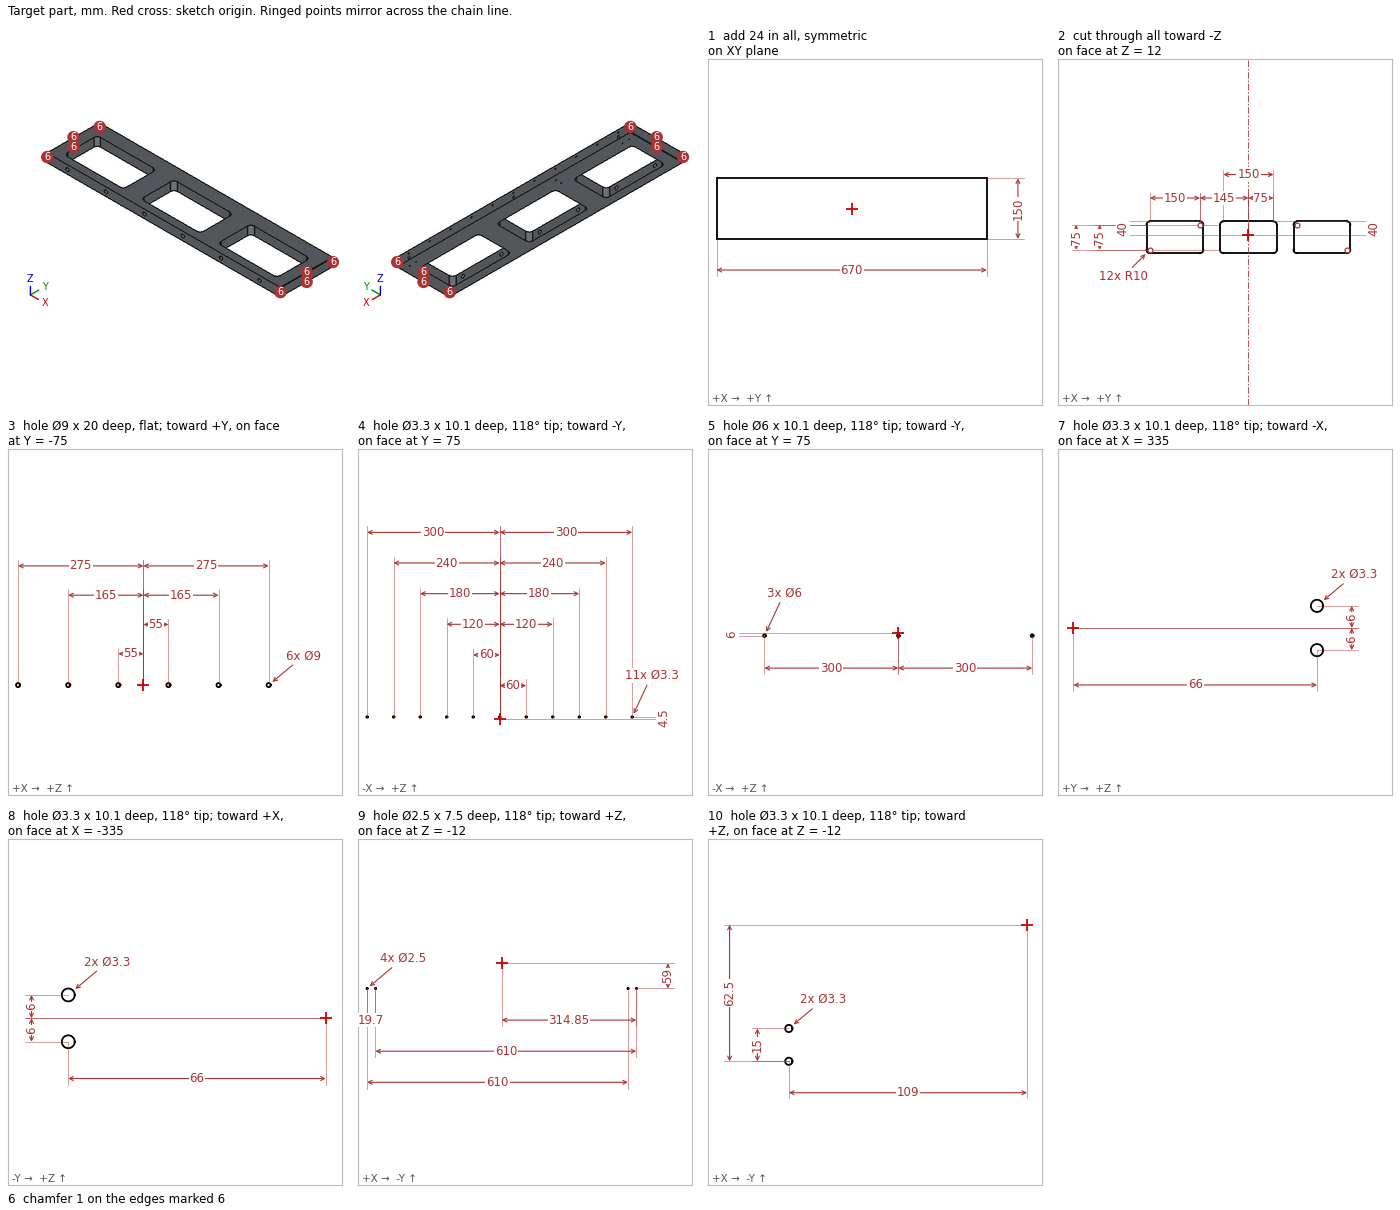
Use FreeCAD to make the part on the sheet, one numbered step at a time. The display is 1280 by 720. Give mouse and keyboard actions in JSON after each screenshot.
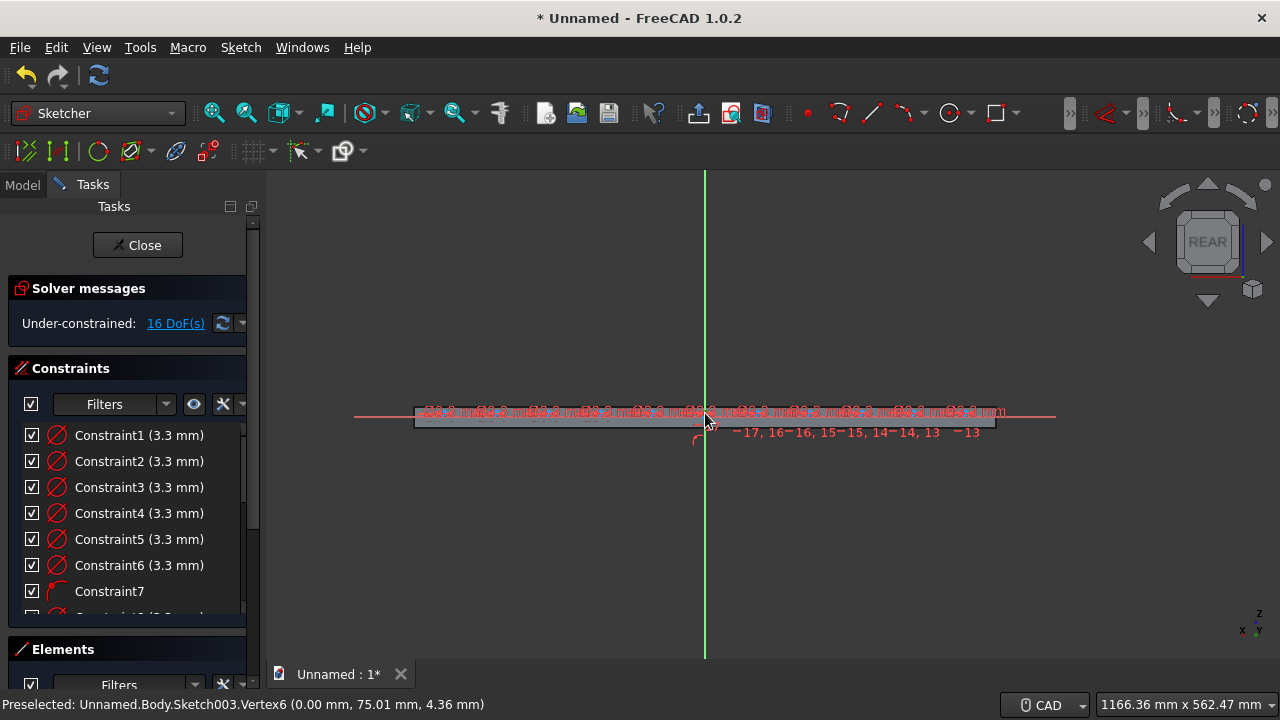
{"action": "left_click", "coordinate": [653, 413]}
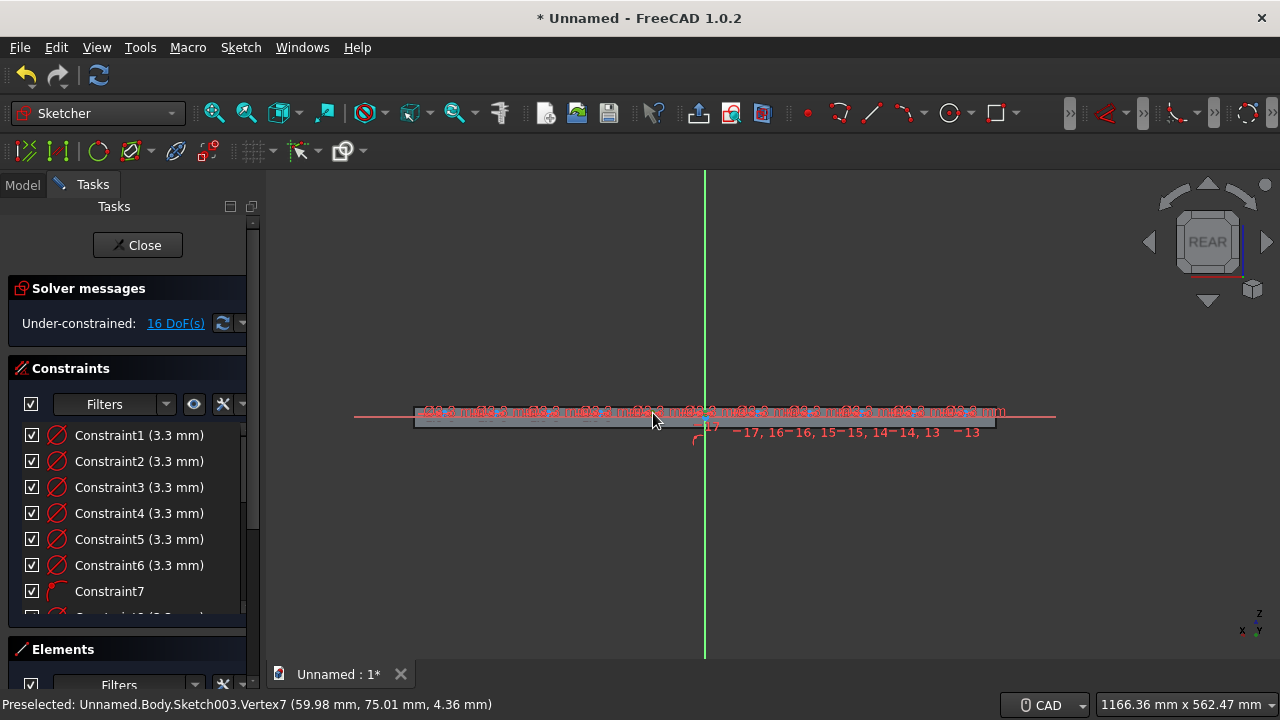
{"action": "key", "text": "h"}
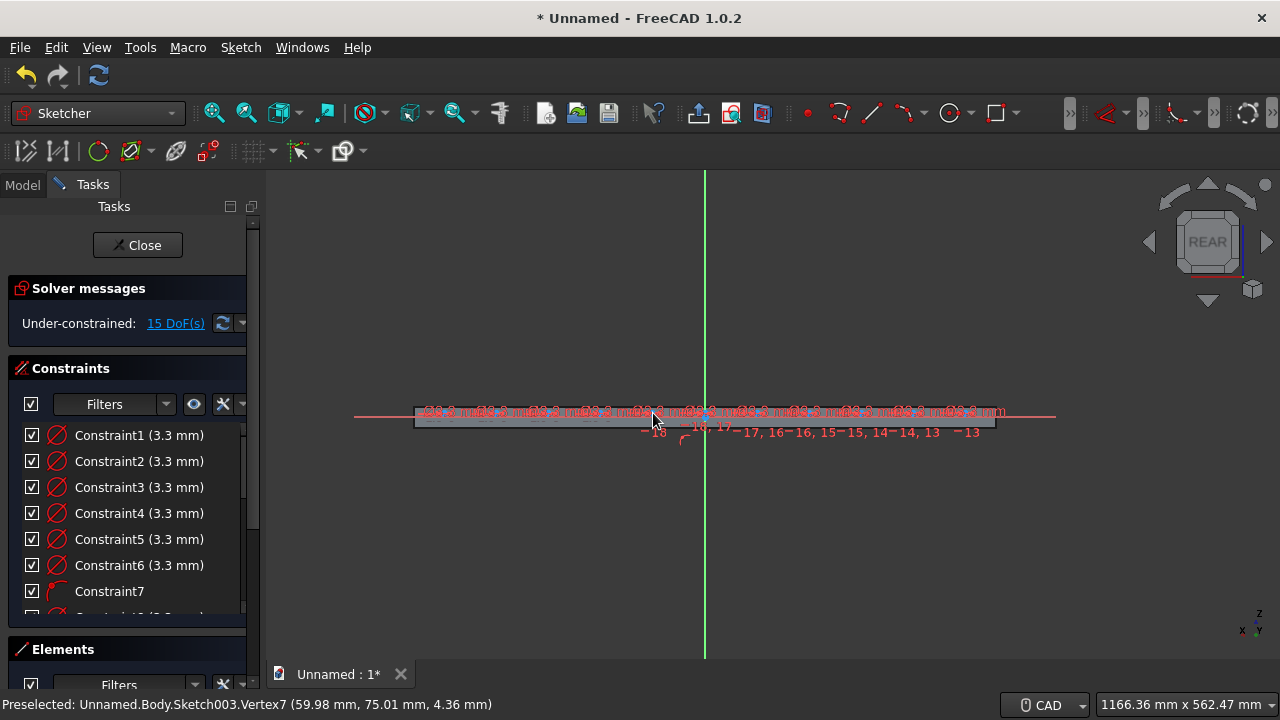
{"action": "left_click", "coordinate": [653, 413]}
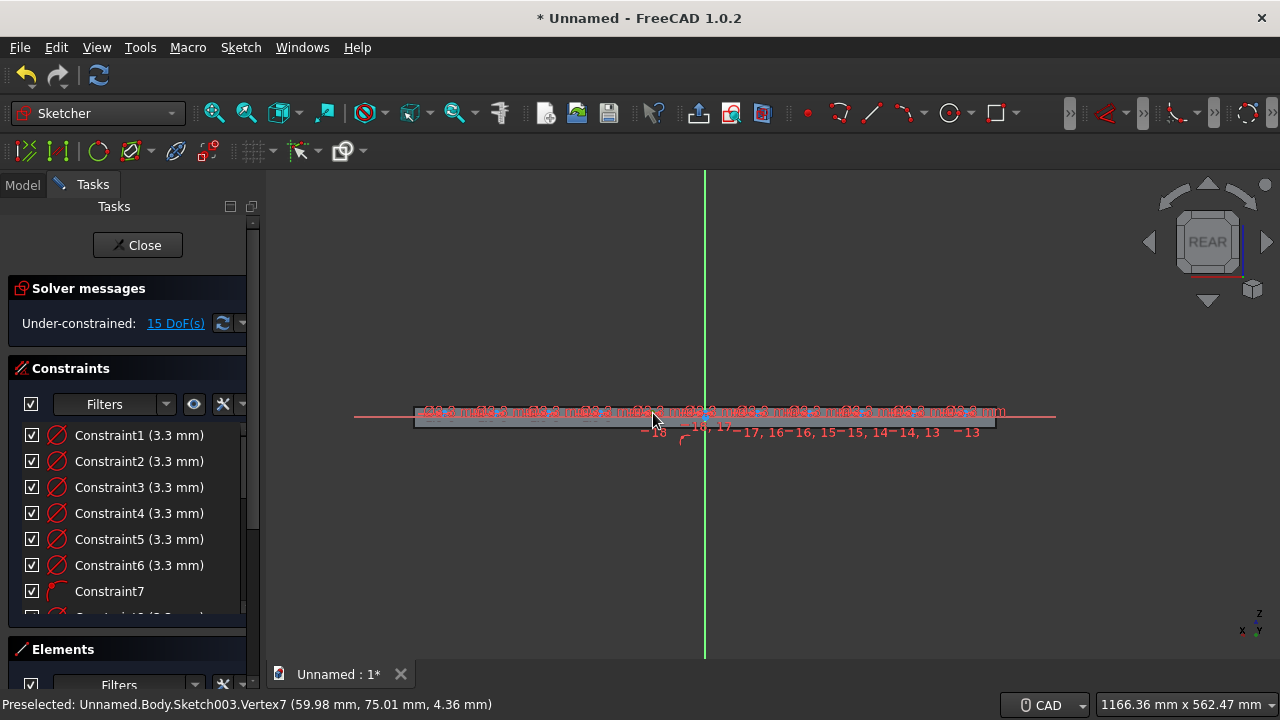
{"action": "left_click", "coordinate": [601, 414]}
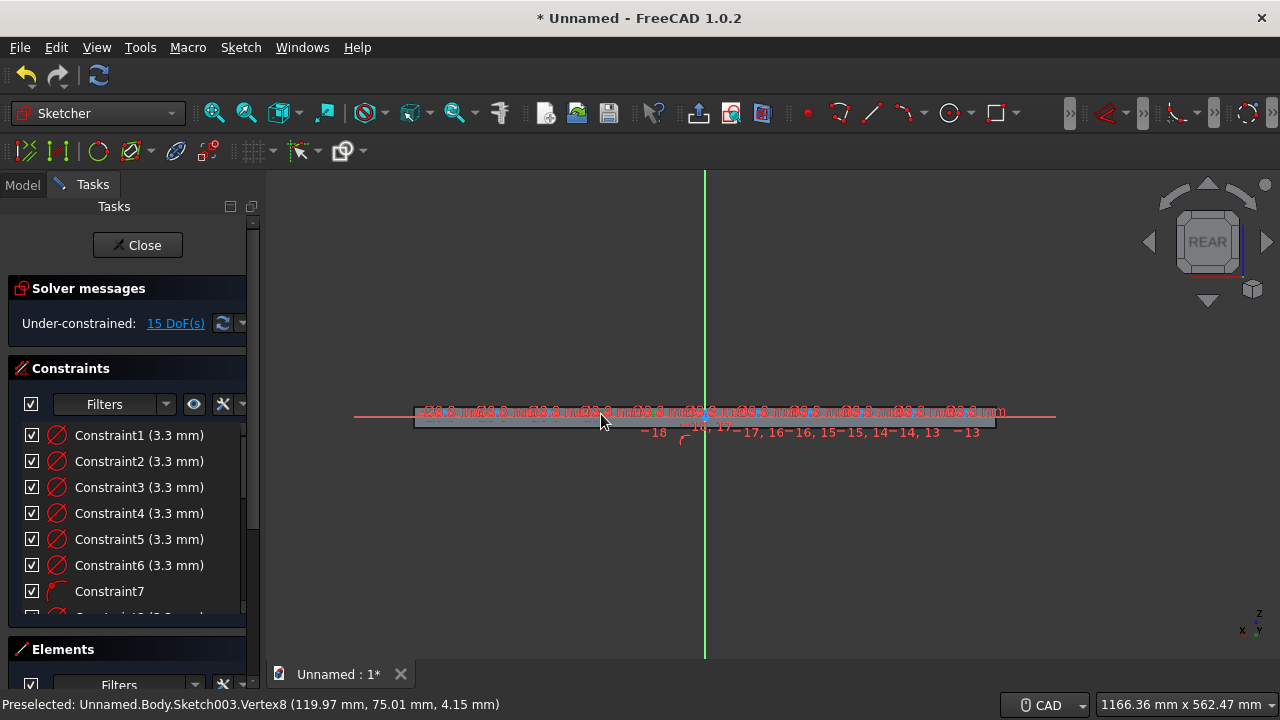
{"action": "key", "text": "h"}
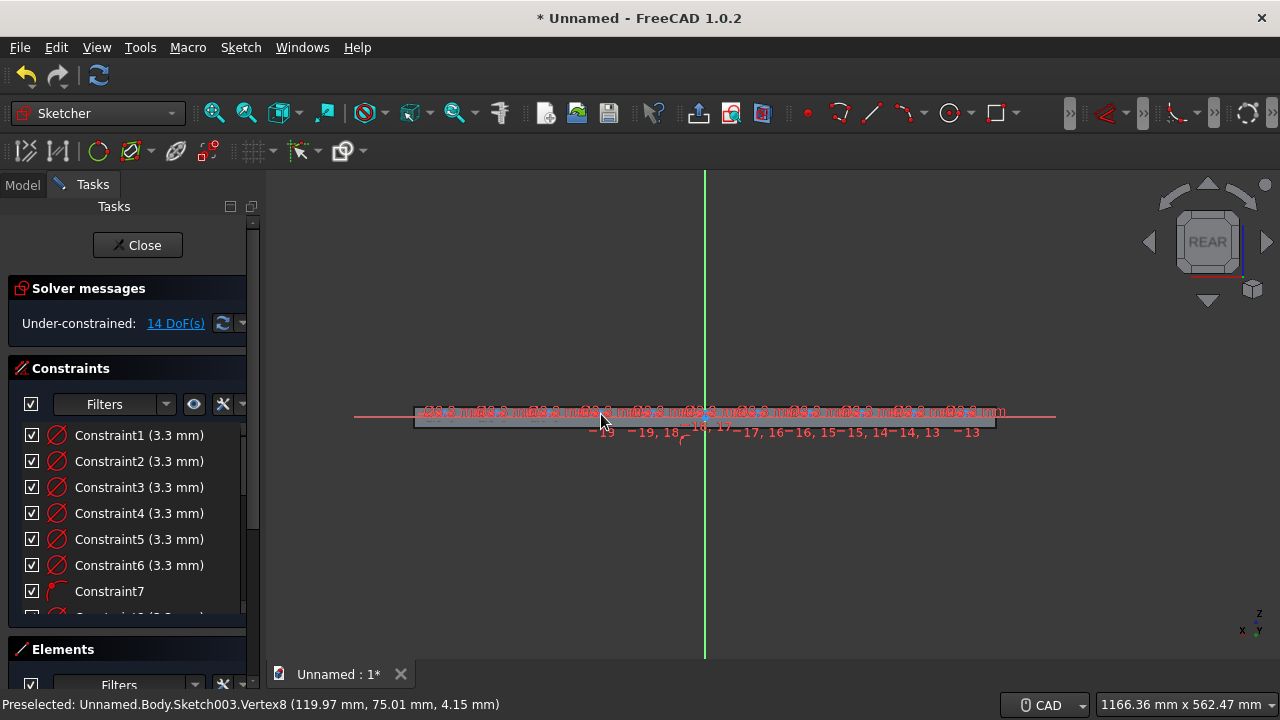
{"action": "left_click", "coordinate": [601, 413]}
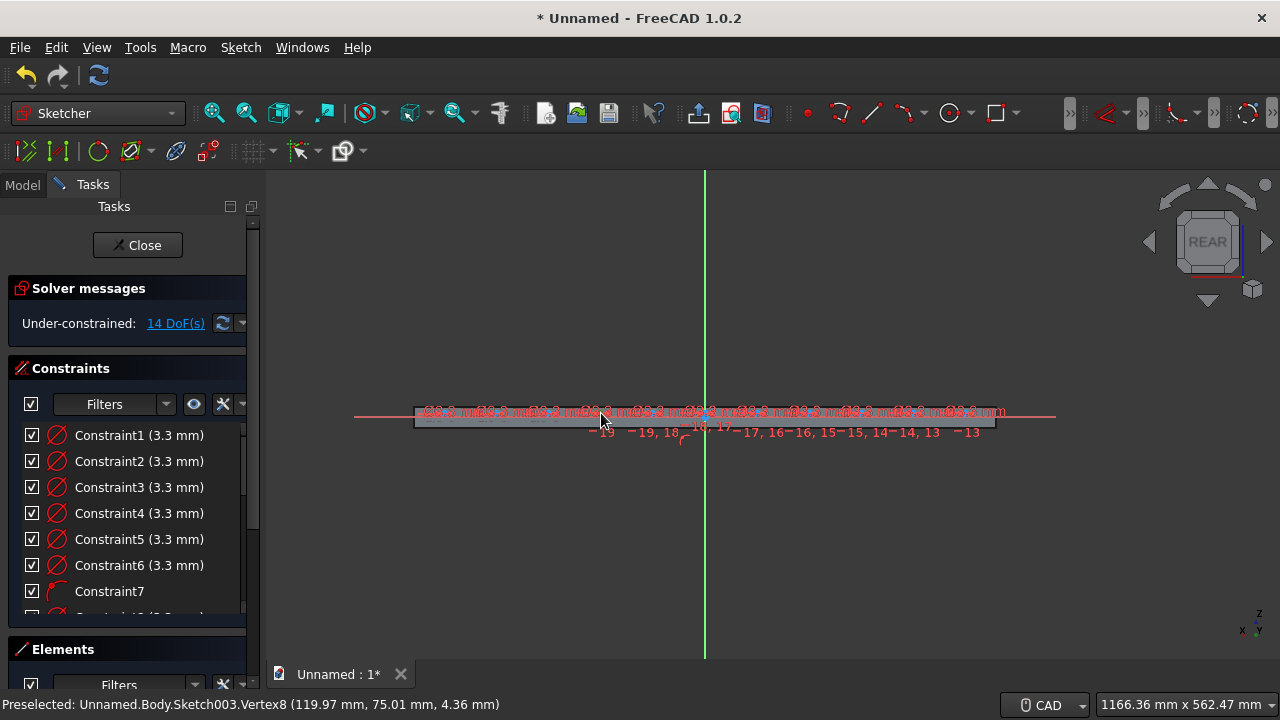
{"action": "left_click", "coordinate": [549, 414]}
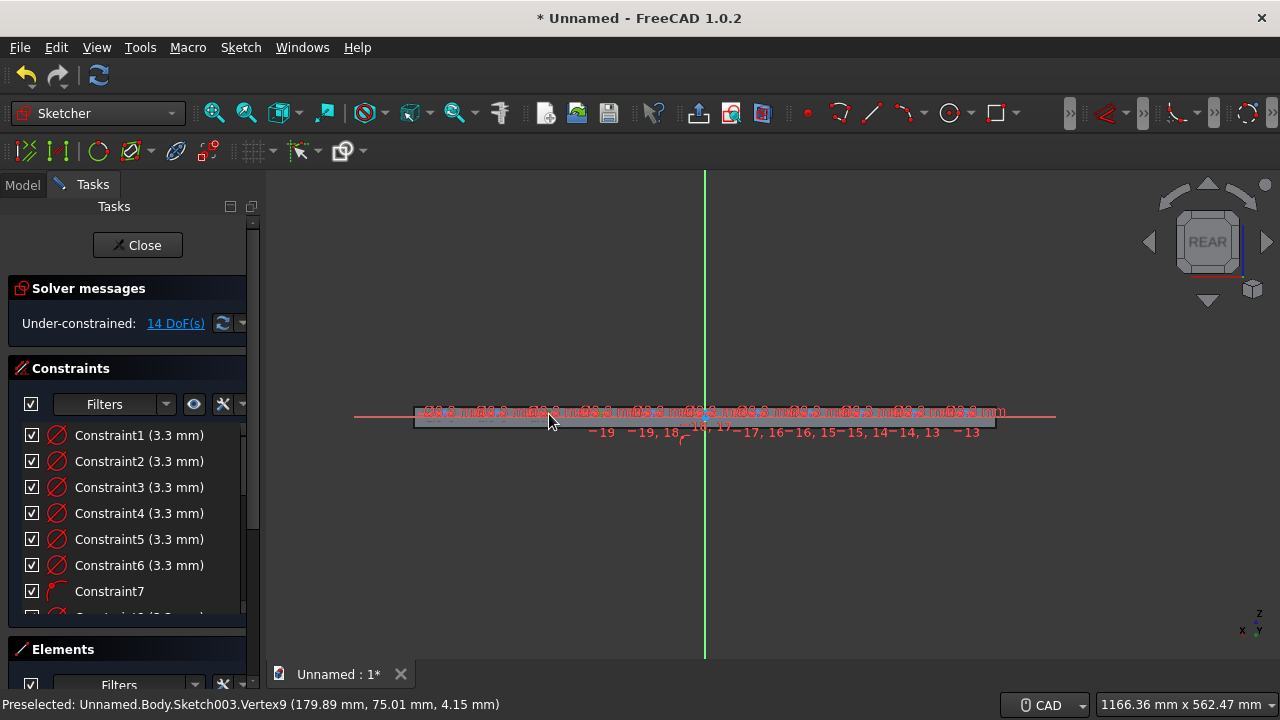
{"action": "key", "text": "h"}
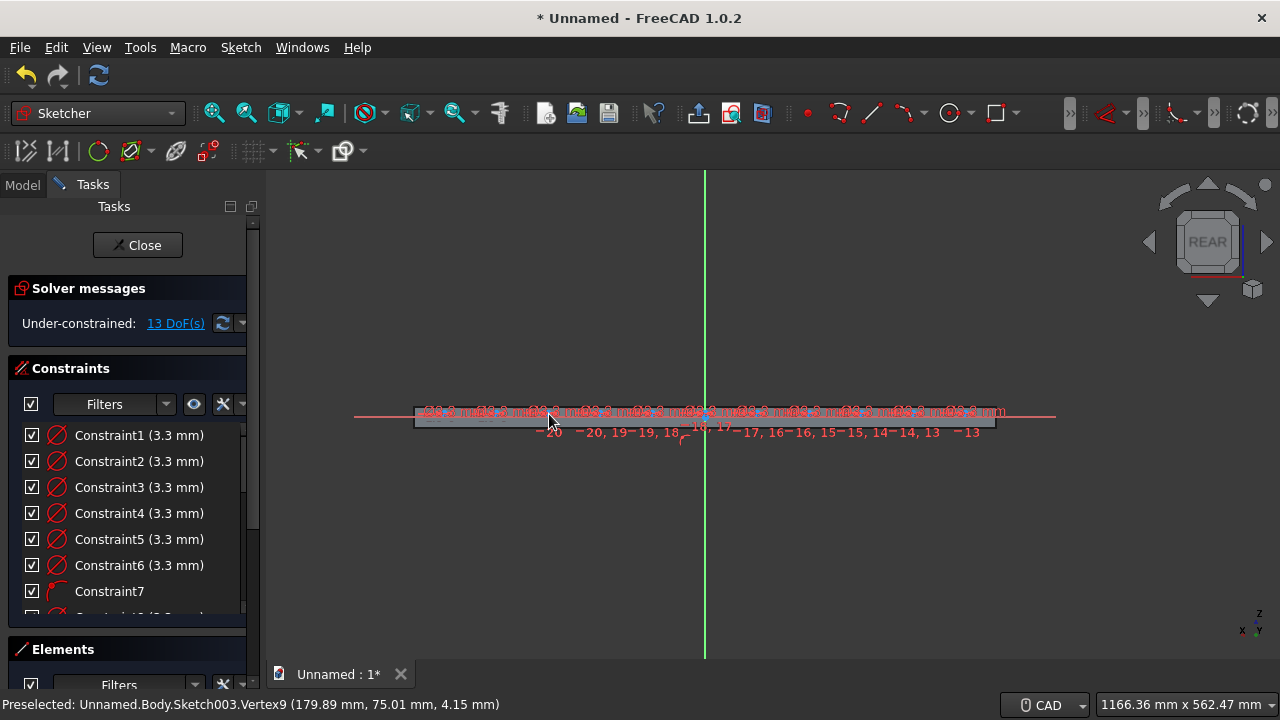
{"action": "left_click", "coordinate": [549, 413]}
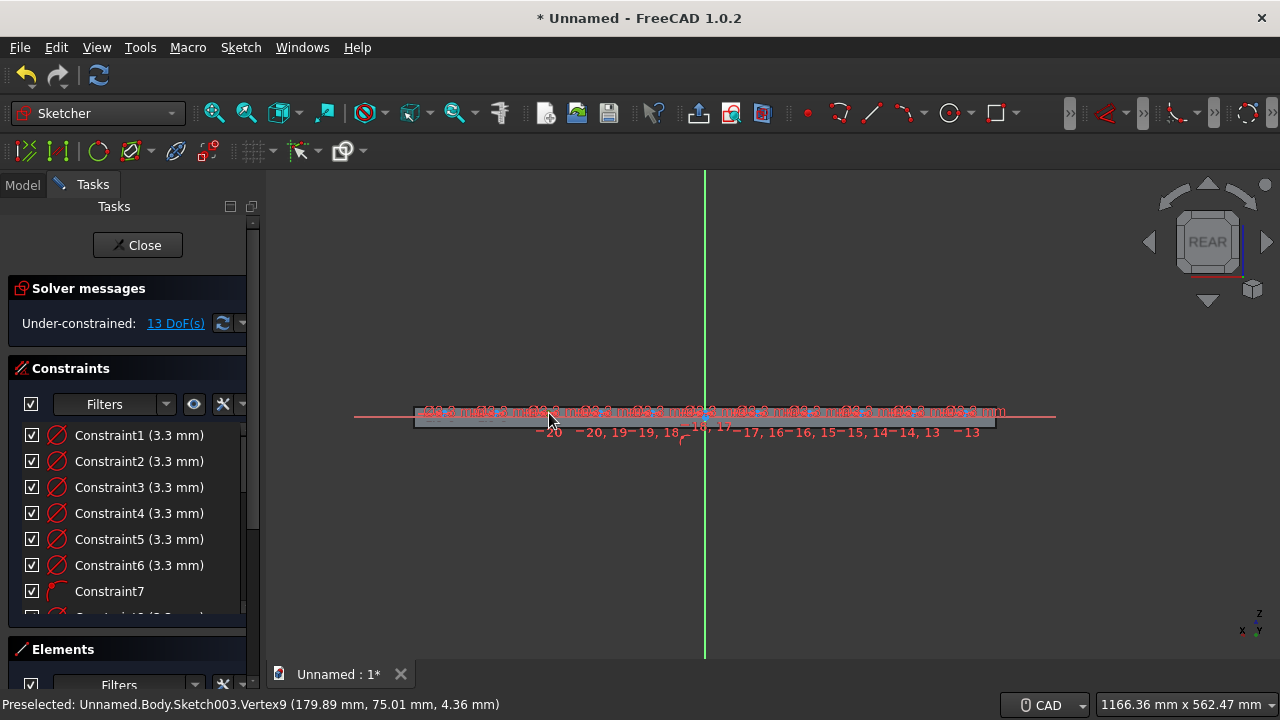
{"action": "left_click", "coordinate": [496, 414]}